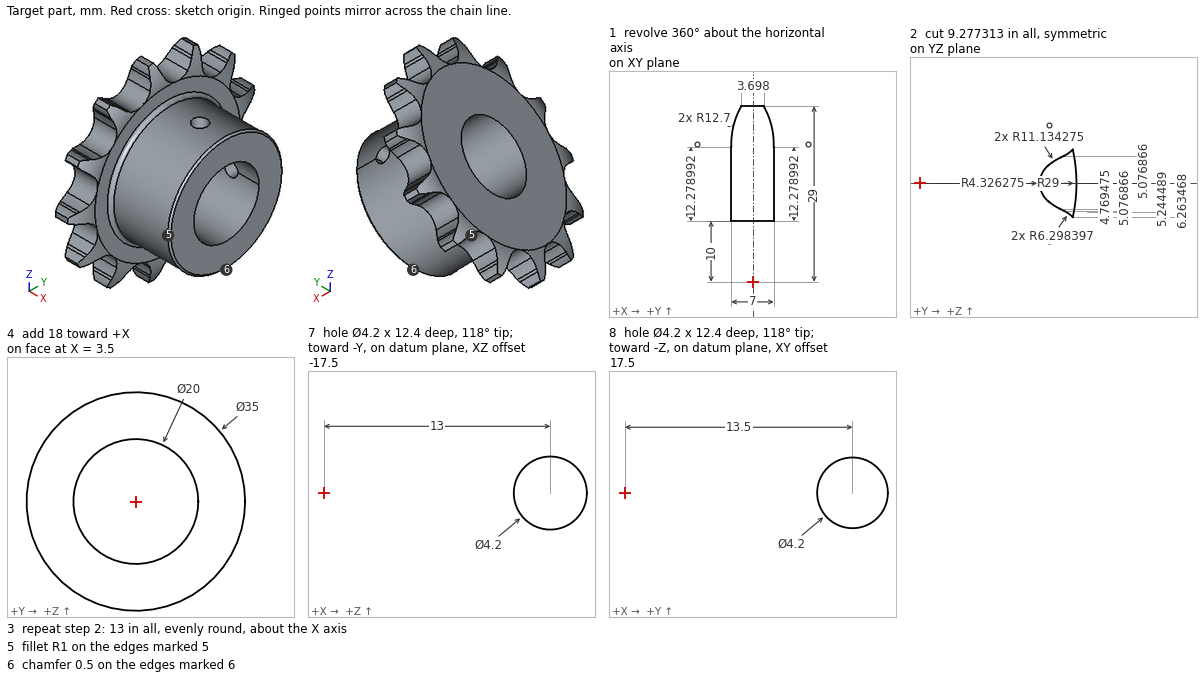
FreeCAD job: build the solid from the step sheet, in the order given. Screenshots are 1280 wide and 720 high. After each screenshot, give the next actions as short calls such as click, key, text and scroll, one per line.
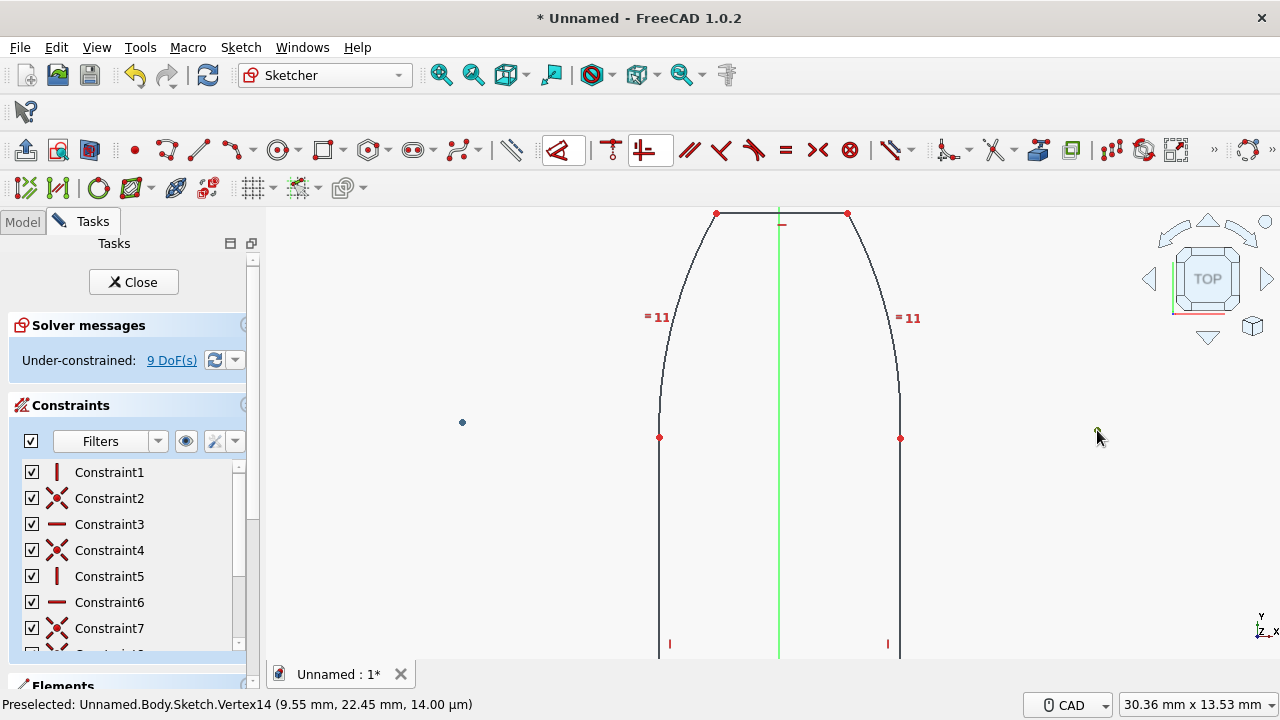
click(779, 603)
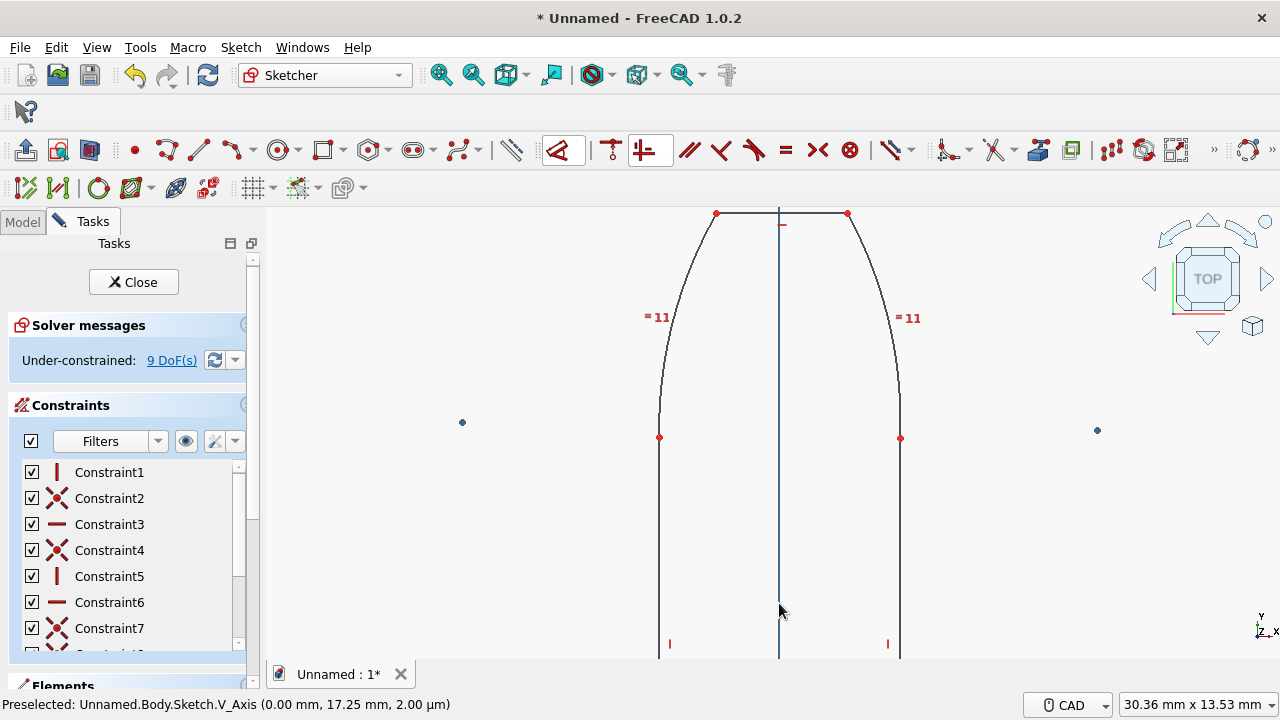
click(818, 150)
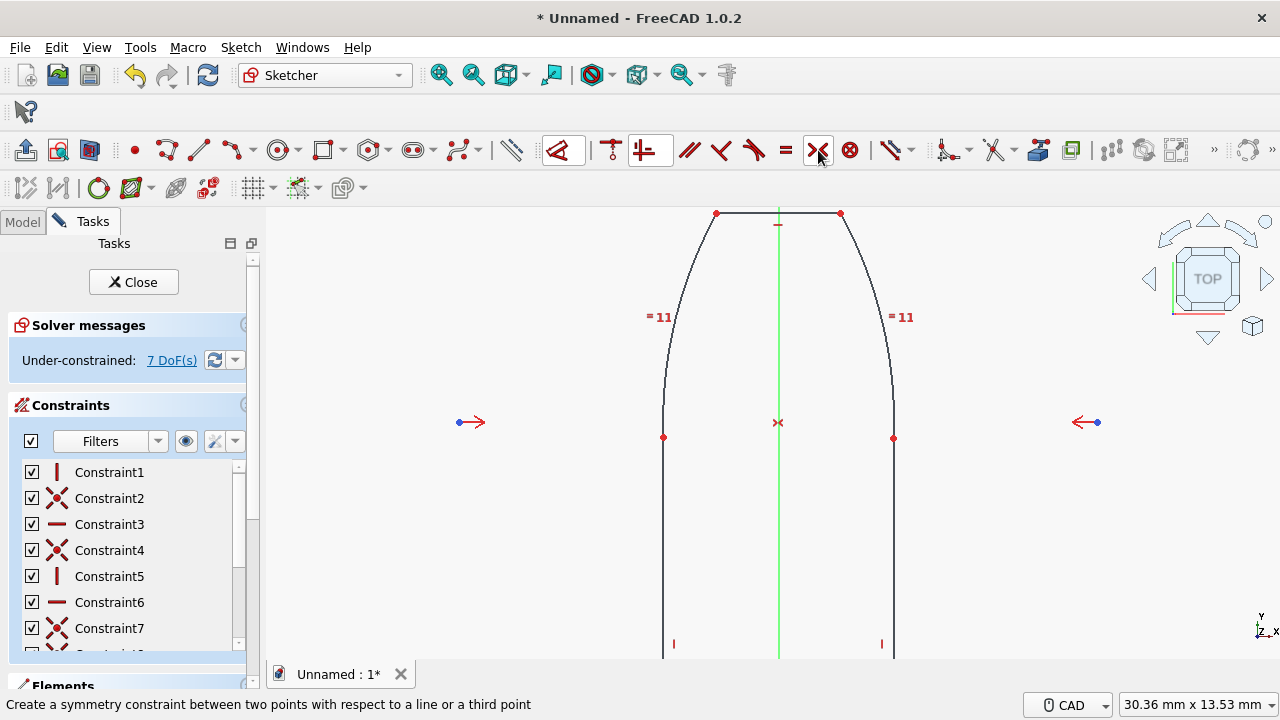
click(558, 150)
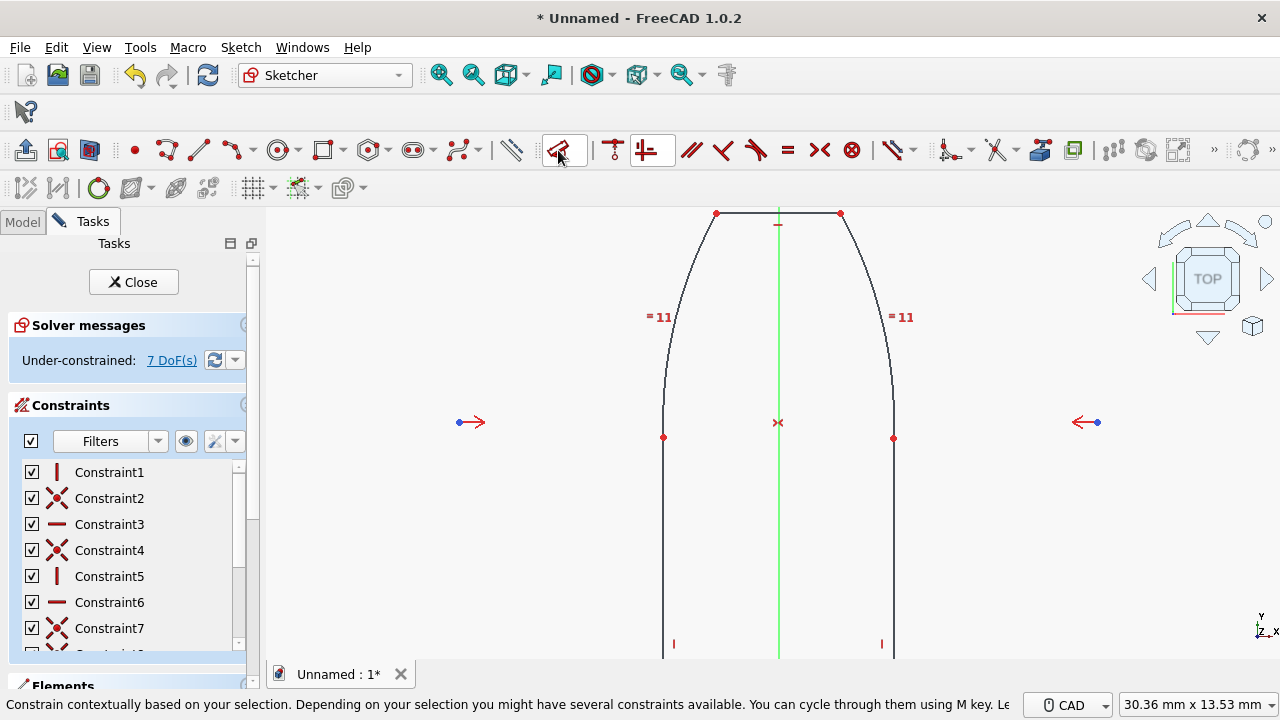
click(891, 368)
click(923, 364)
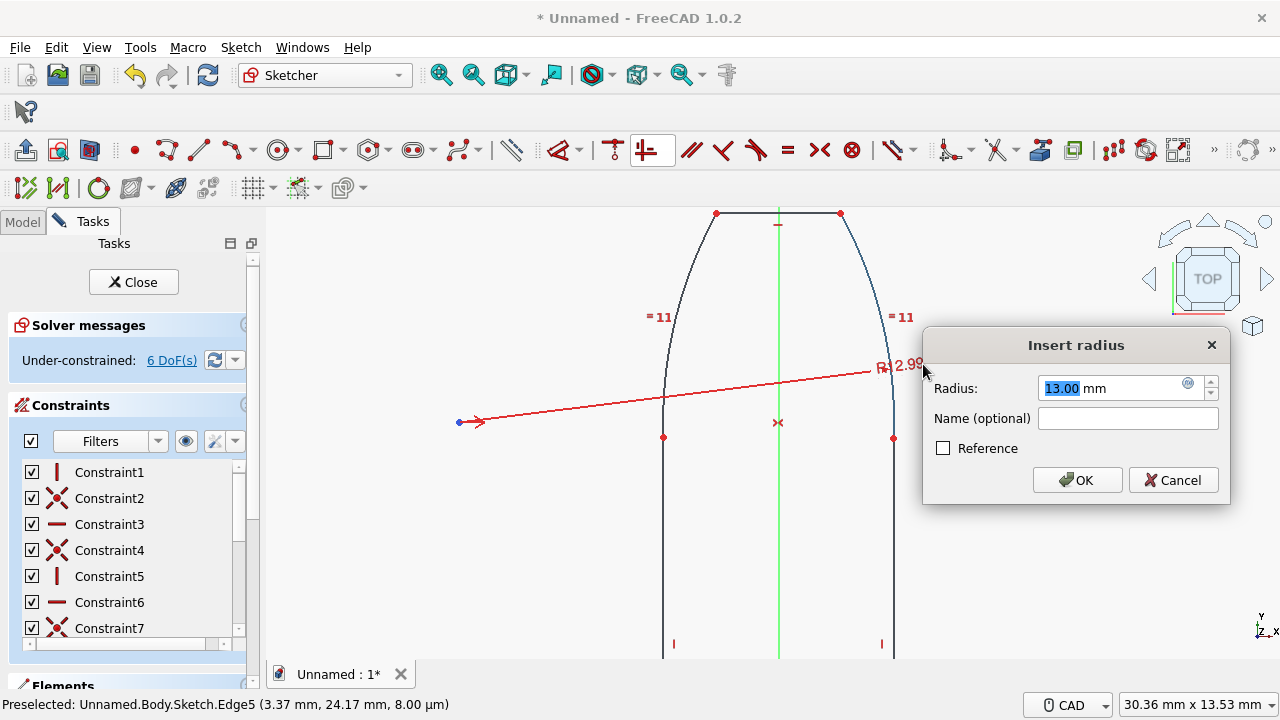
text(12.7)
key(Return)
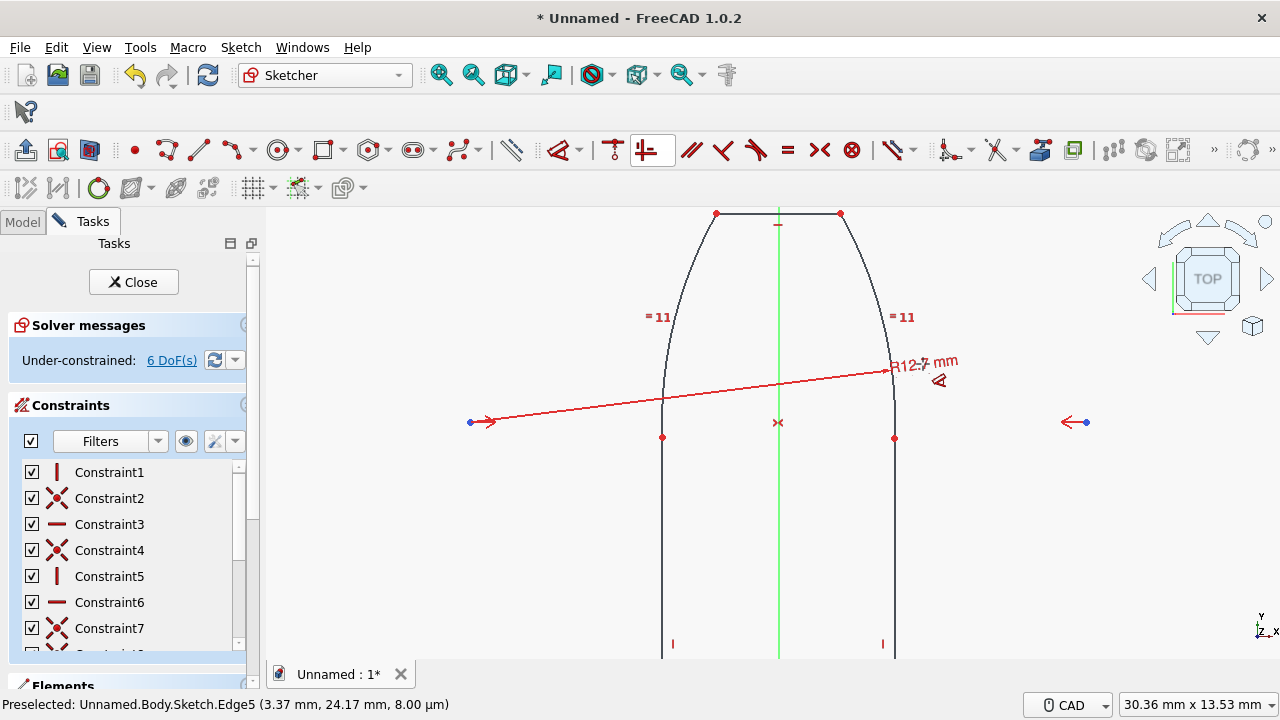
scroll(673, 320, down, 6)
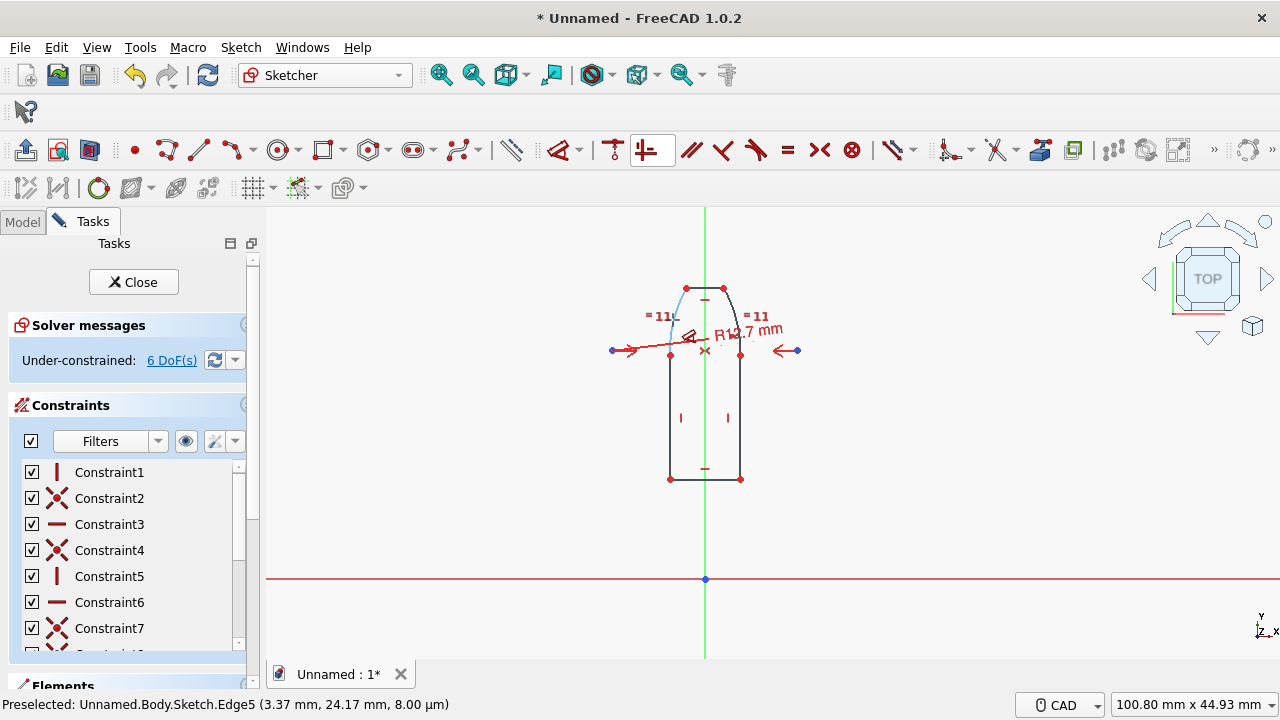
click(691, 480)
click(689, 514)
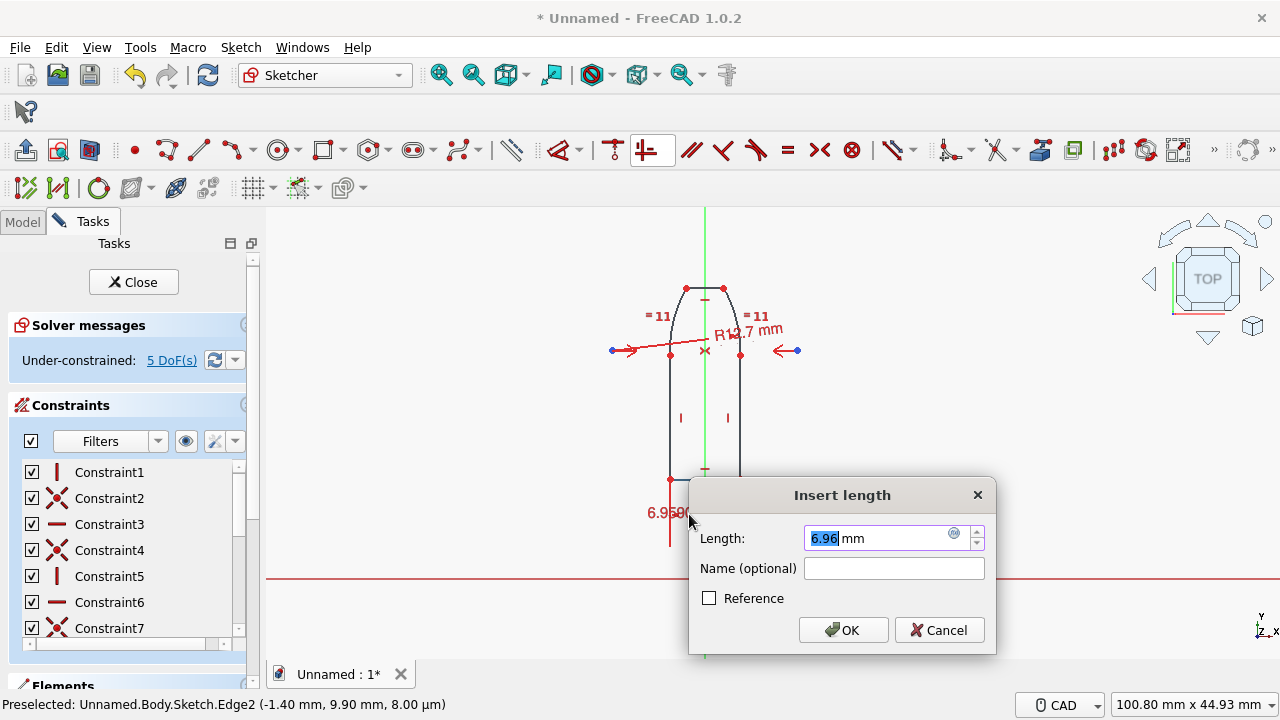
text(7)
key(Return)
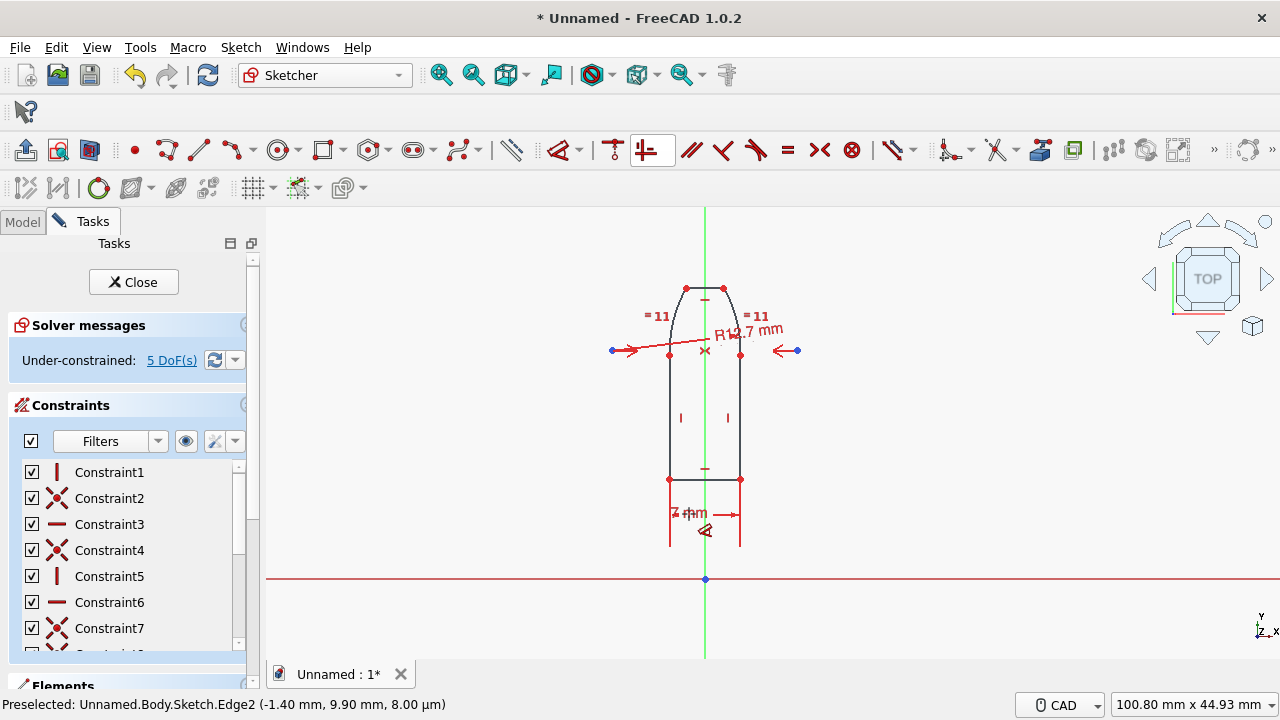
click(670, 480)
click(636, 552)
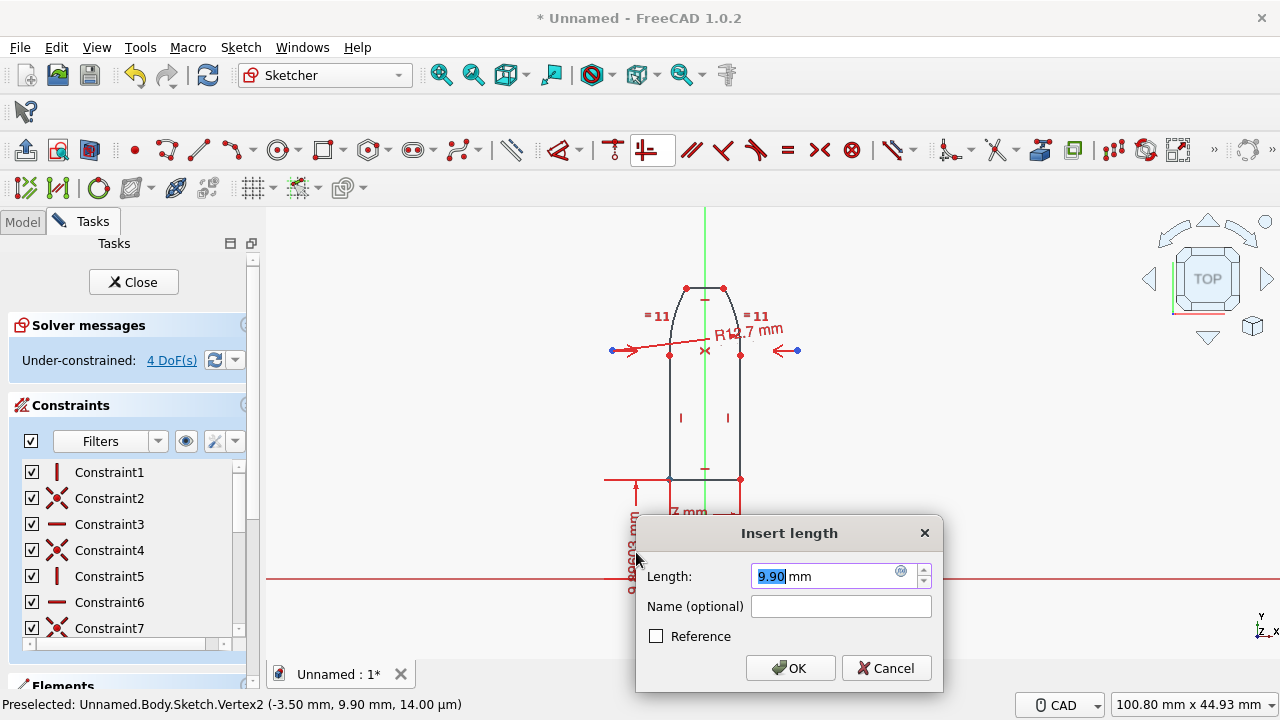
text(10)
key(Return)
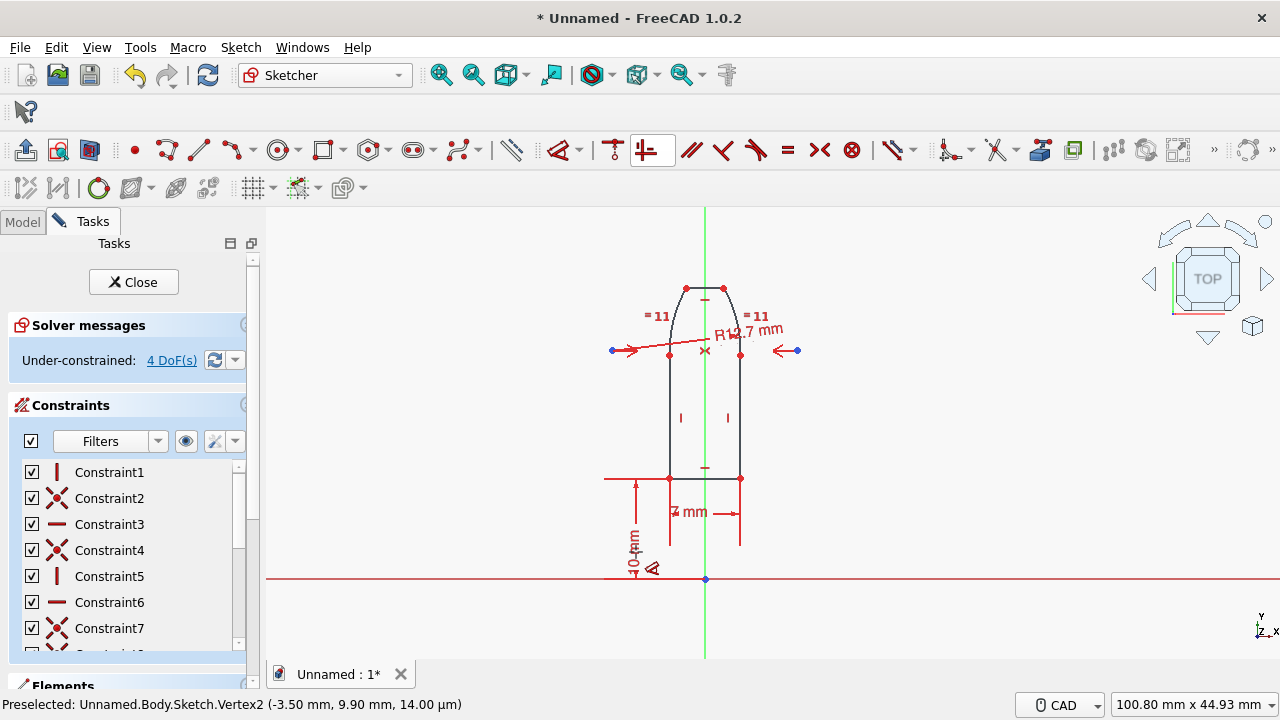
click(724, 288)
click(758, 434)